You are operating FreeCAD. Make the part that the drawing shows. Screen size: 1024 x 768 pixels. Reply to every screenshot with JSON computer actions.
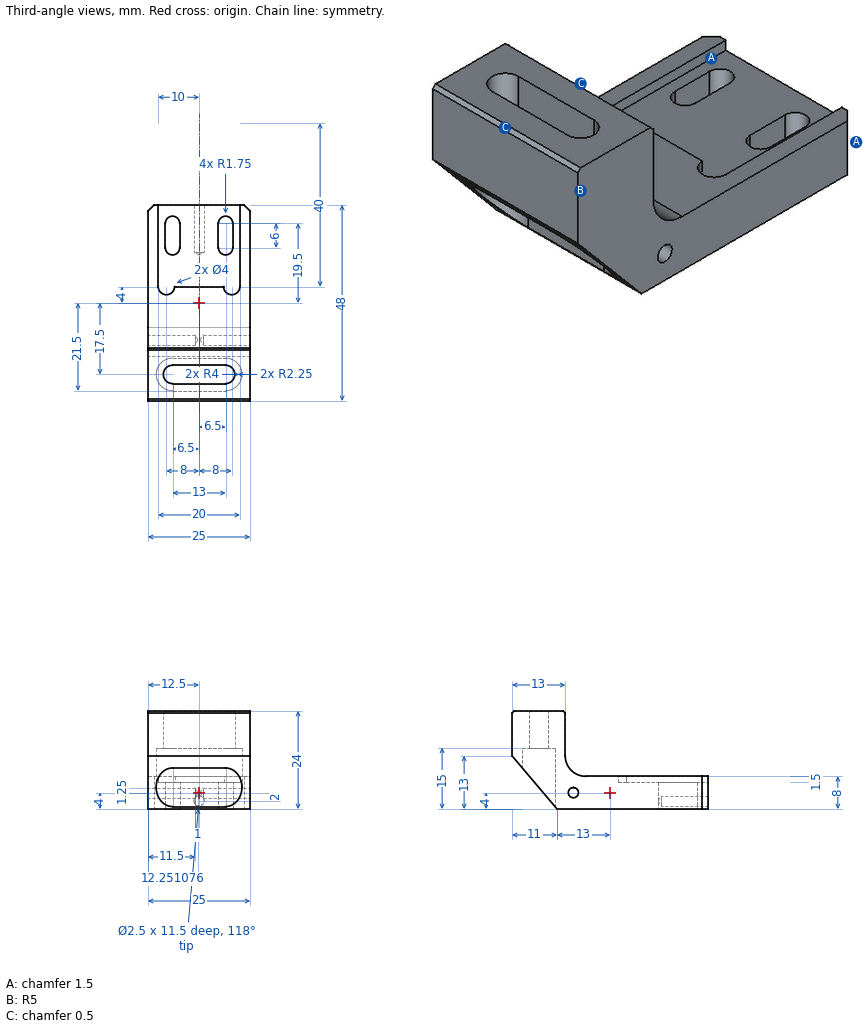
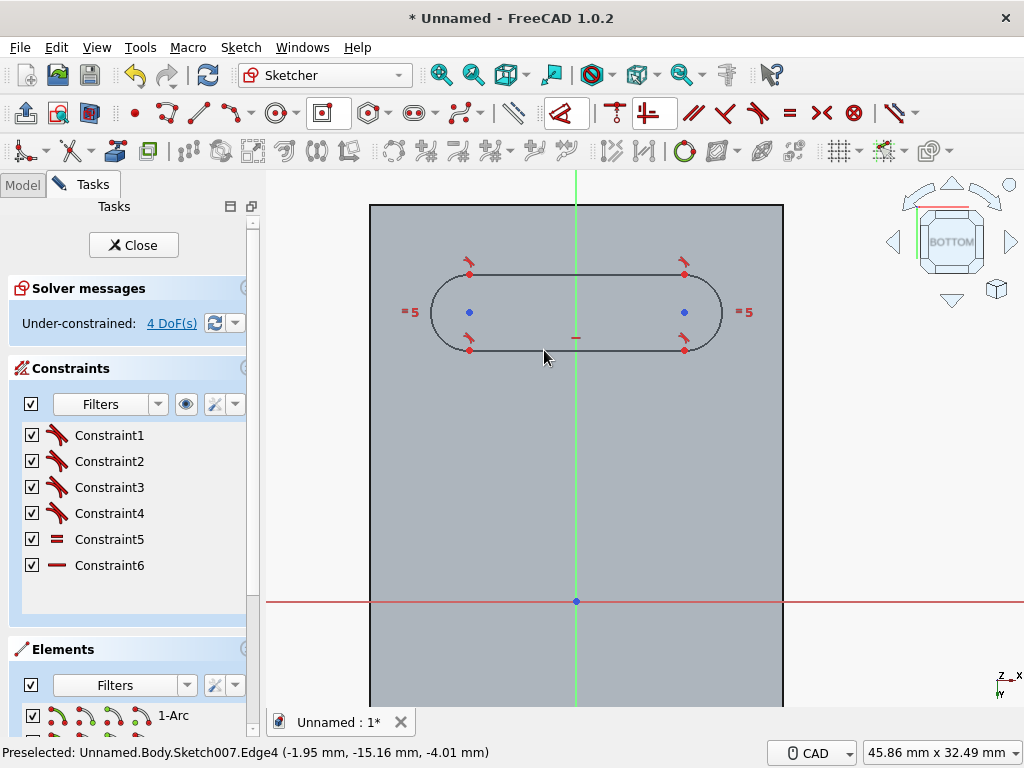
{"action": "left_click", "coordinate": [438, 291]}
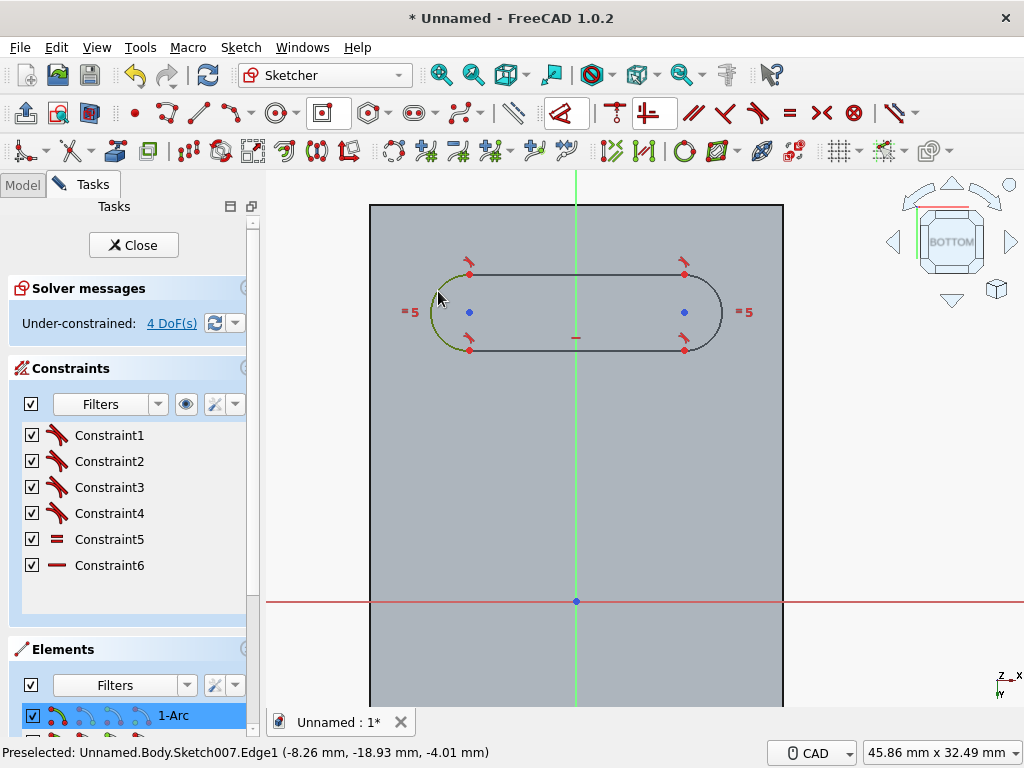
{"action": "left_click", "coordinate": [584, 114]}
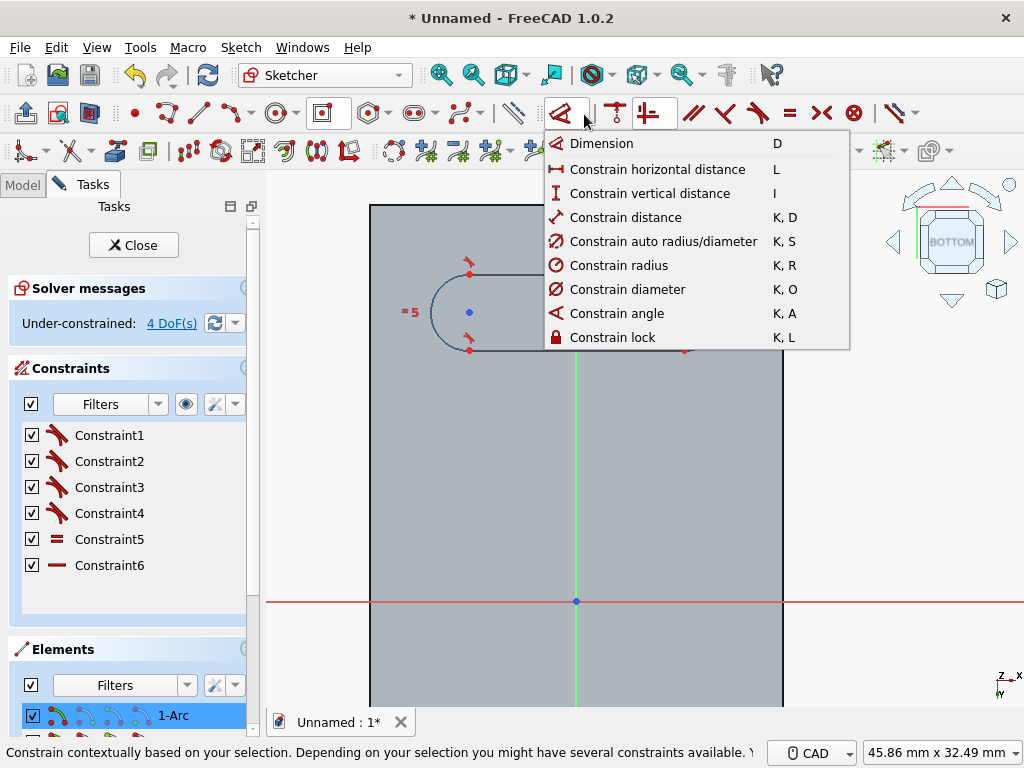
{"action": "left_click", "coordinate": [697, 265]}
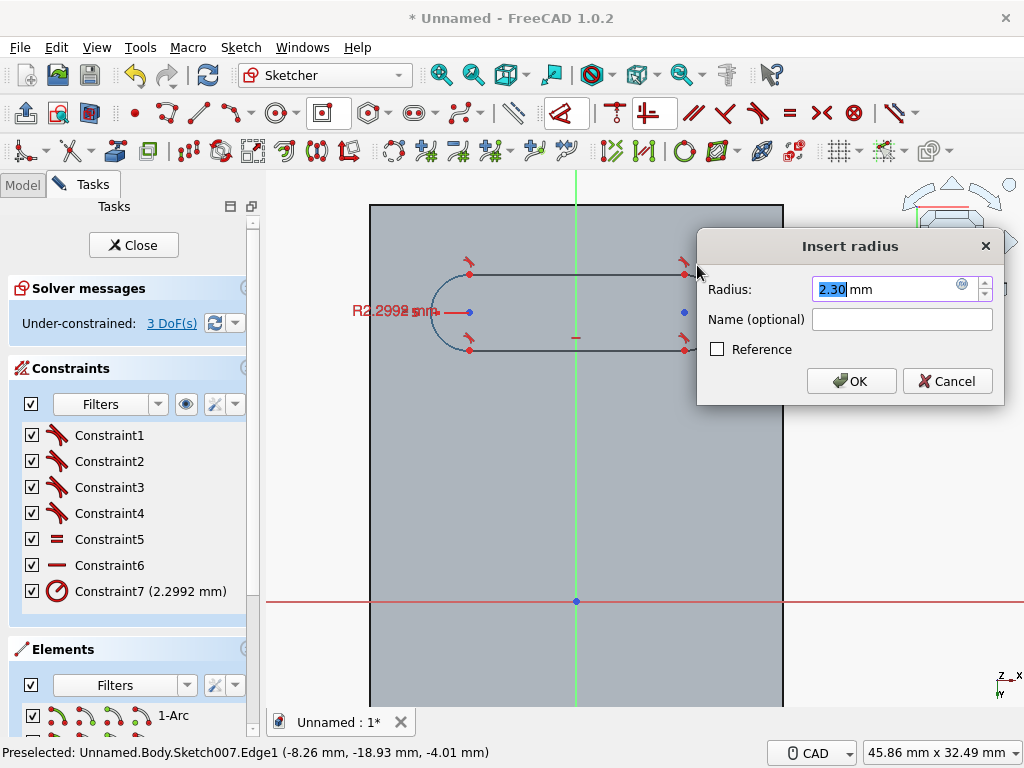
{"action": "type", "text": "2.25"}
{"action": "key", "text": "Return"}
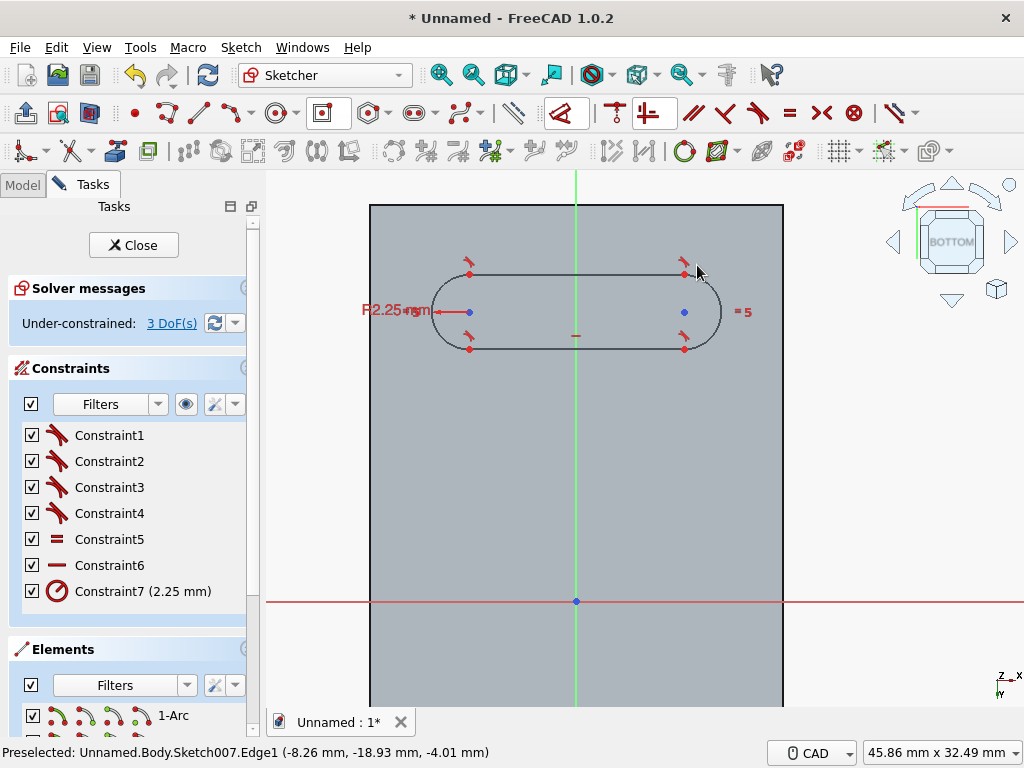
{"action": "left_click", "coordinate": [534, 275]}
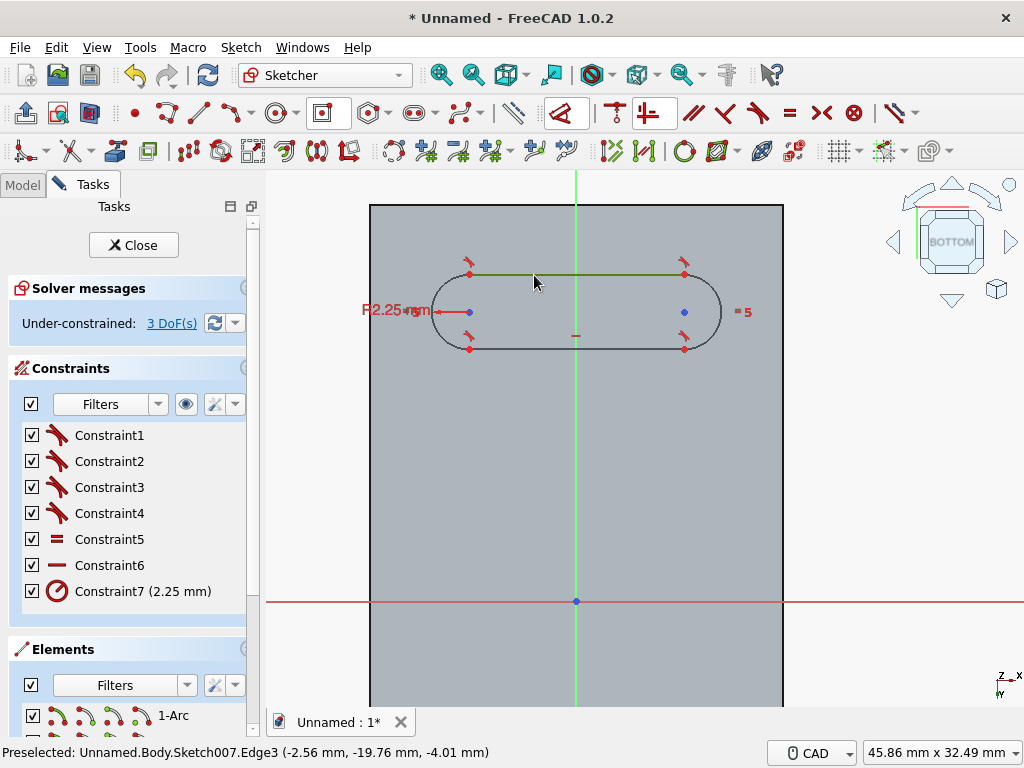
{"action": "left_click", "coordinate": [584, 114]}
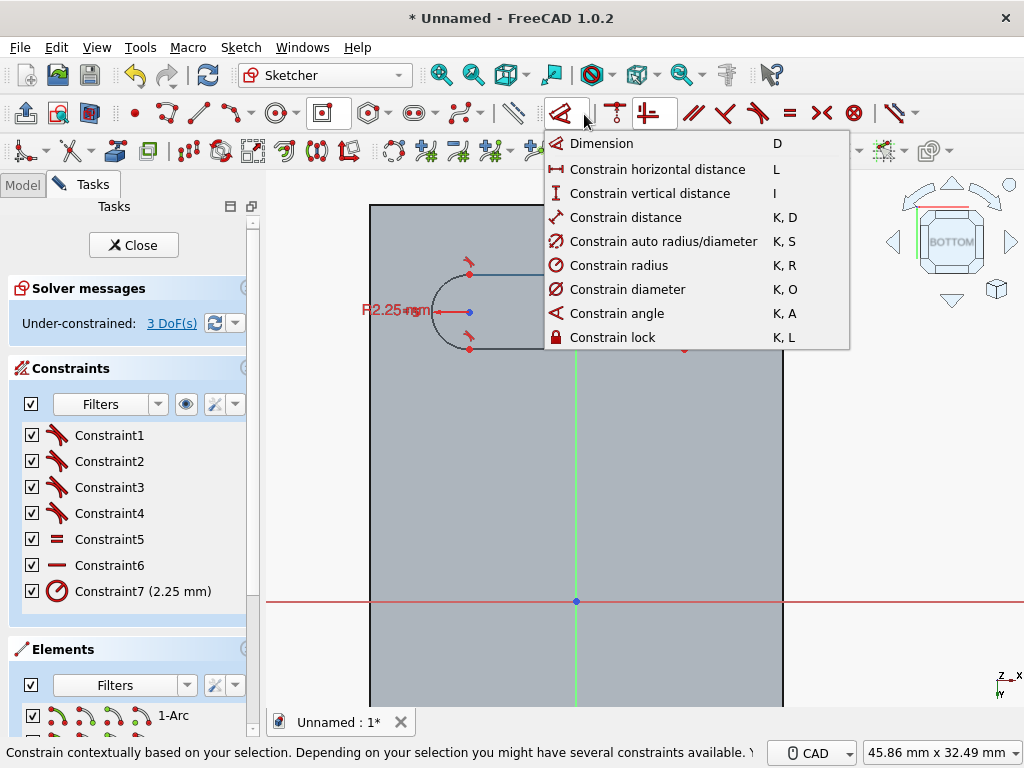
{"action": "left_click", "coordinate": [697, 169]}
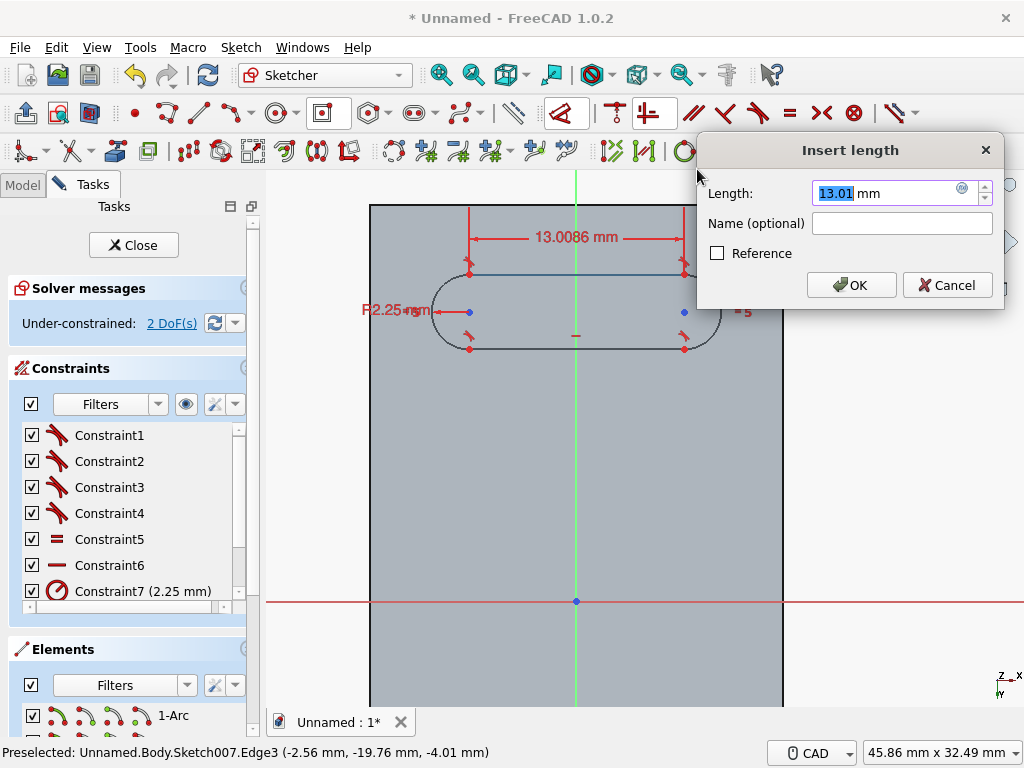
{"action": "type", "text": "13"}
{"action": "key", "text": "Return"}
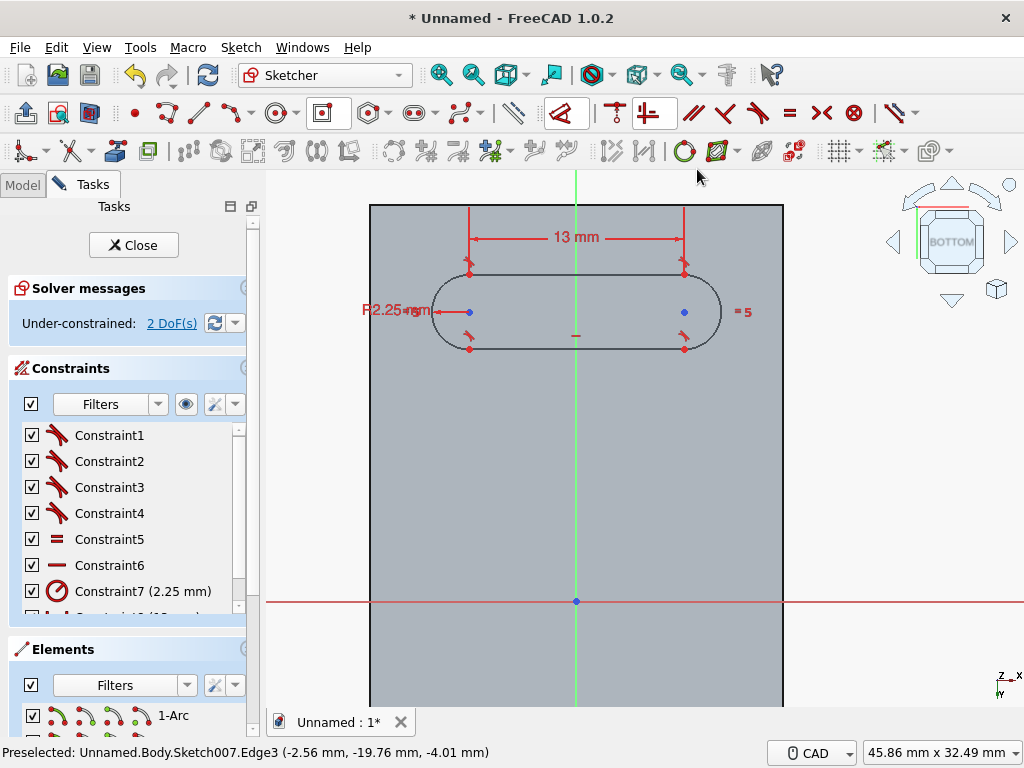
{"action": "left_click", "coordinate": [469, 275]}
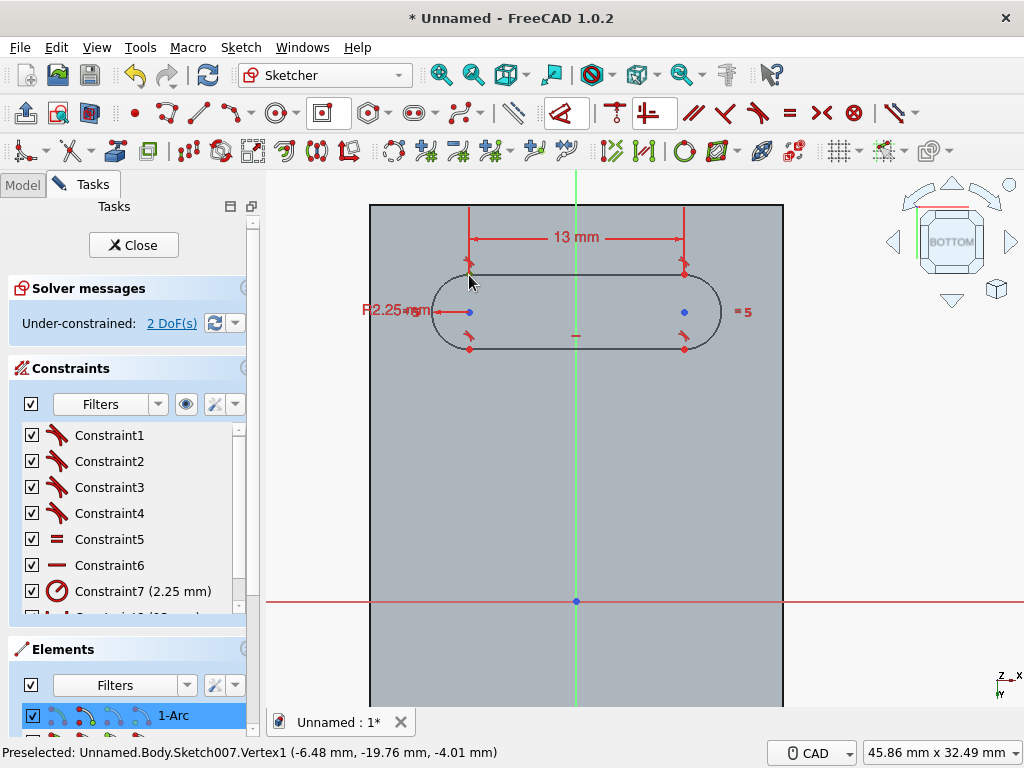
{"action": "key", "text": "l"}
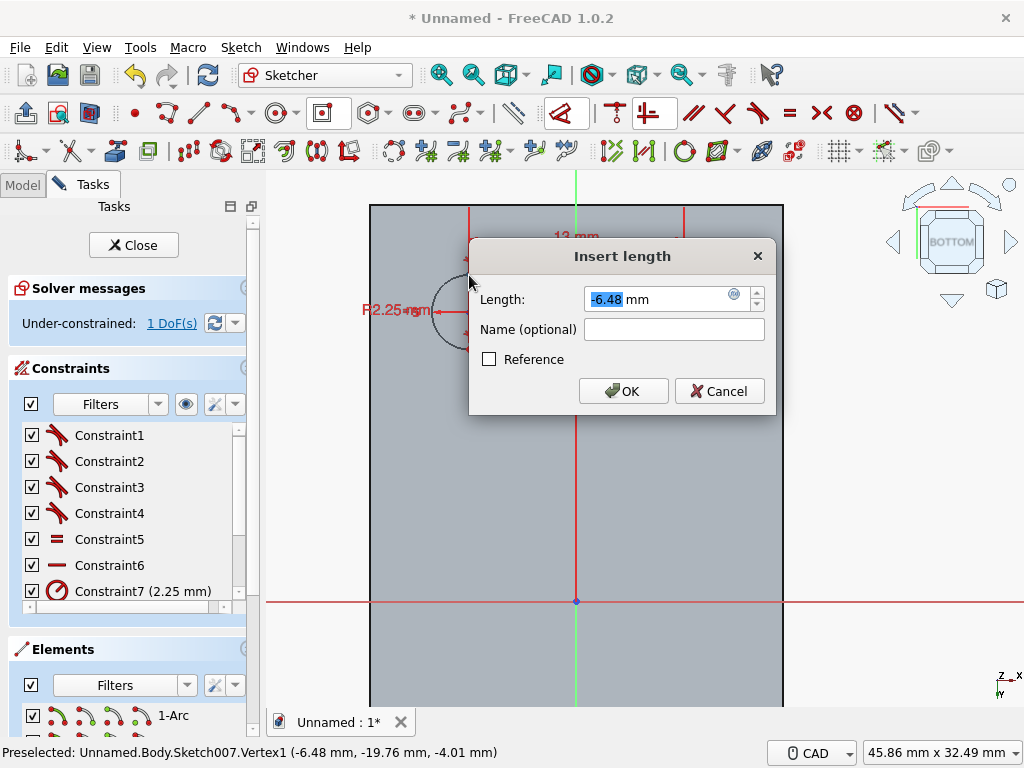
{"action": "type", "text": "-6.5"}
{"action": "key", "text": "Return"}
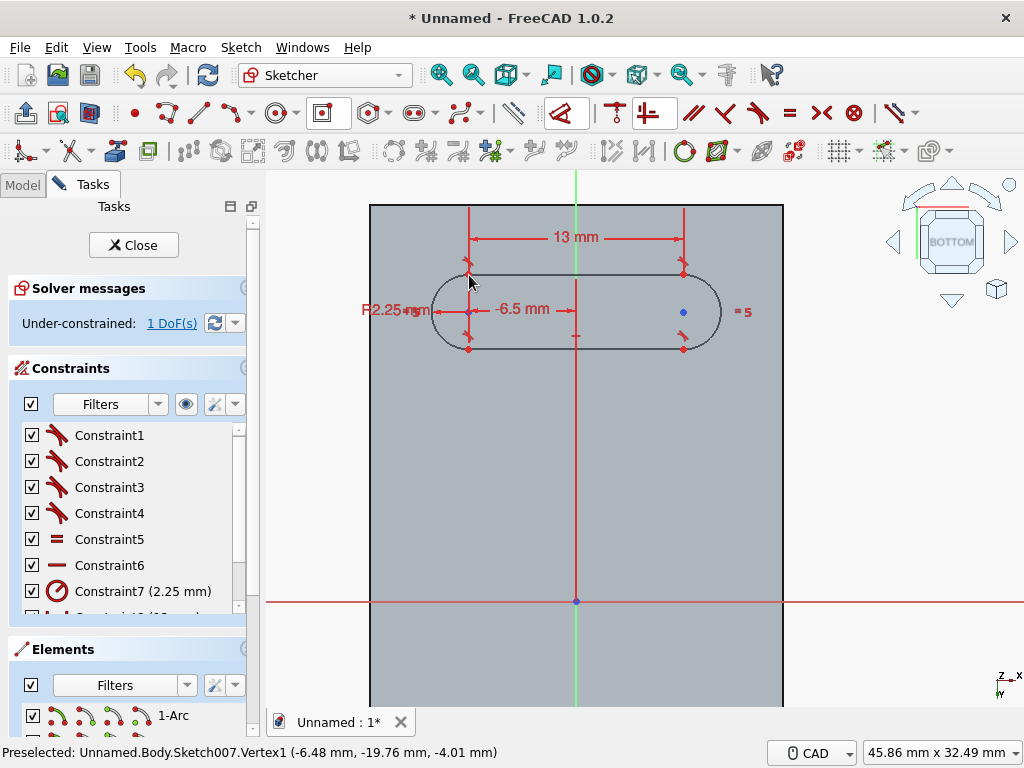
{"action": "left_click", "coordinate": [469, 312]}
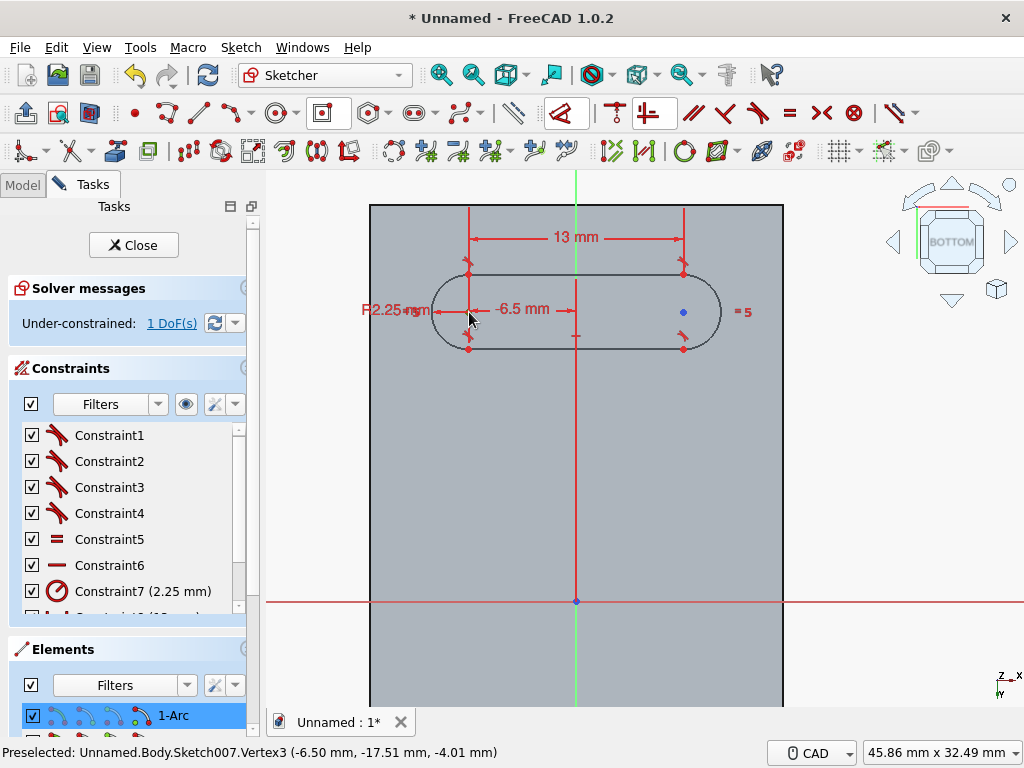
{"action": "left_click", "coordinate": [584, 114]}